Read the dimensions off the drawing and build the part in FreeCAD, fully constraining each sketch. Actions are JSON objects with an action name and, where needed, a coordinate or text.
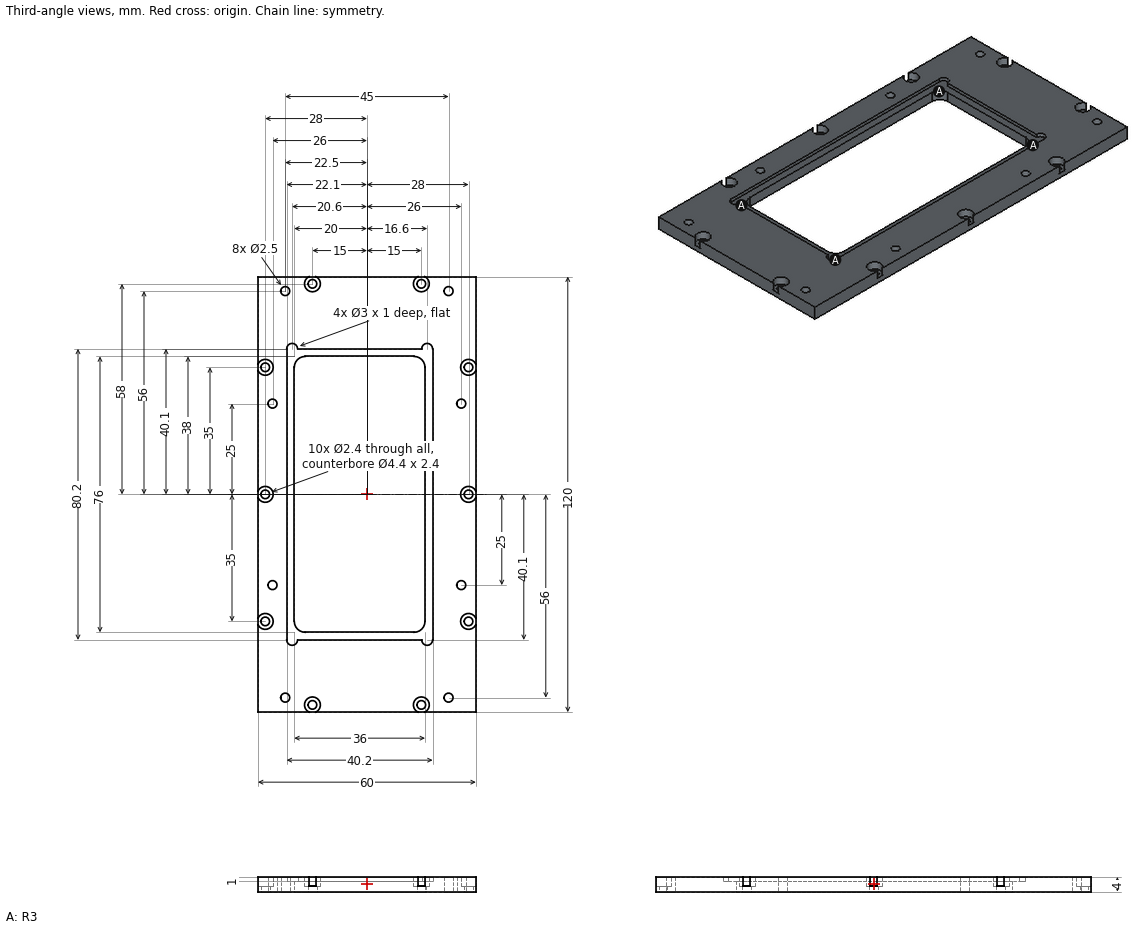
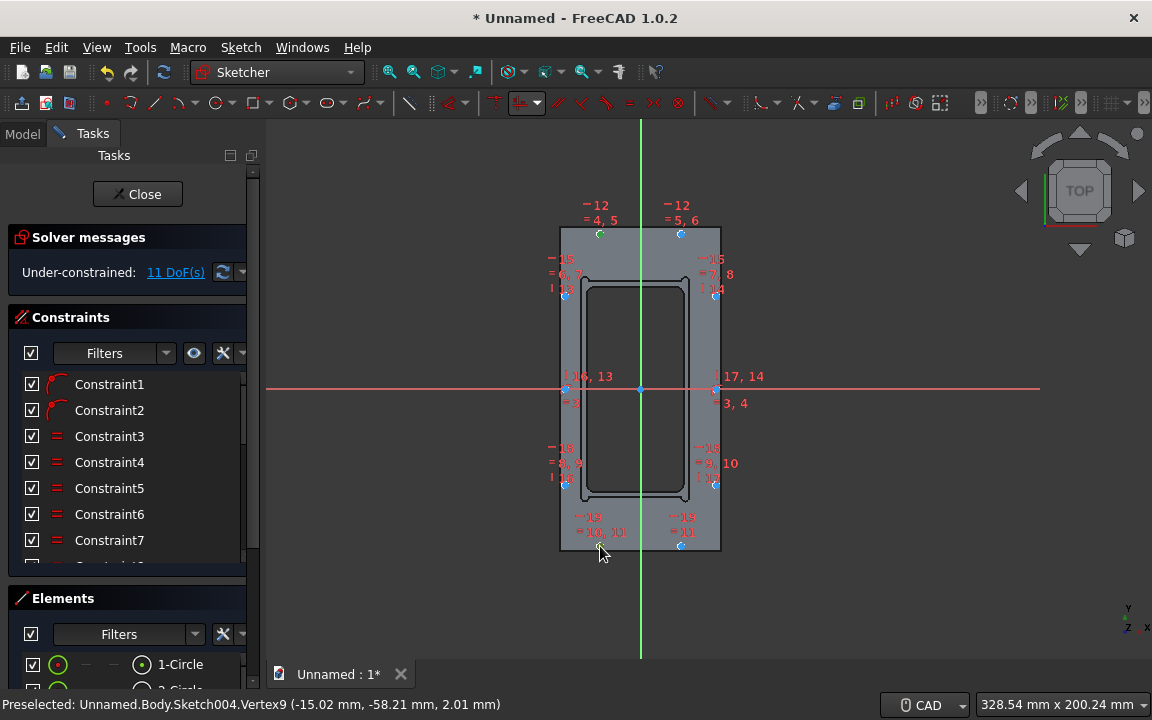
{"action": "left_click", "coordinate": [344, 389]}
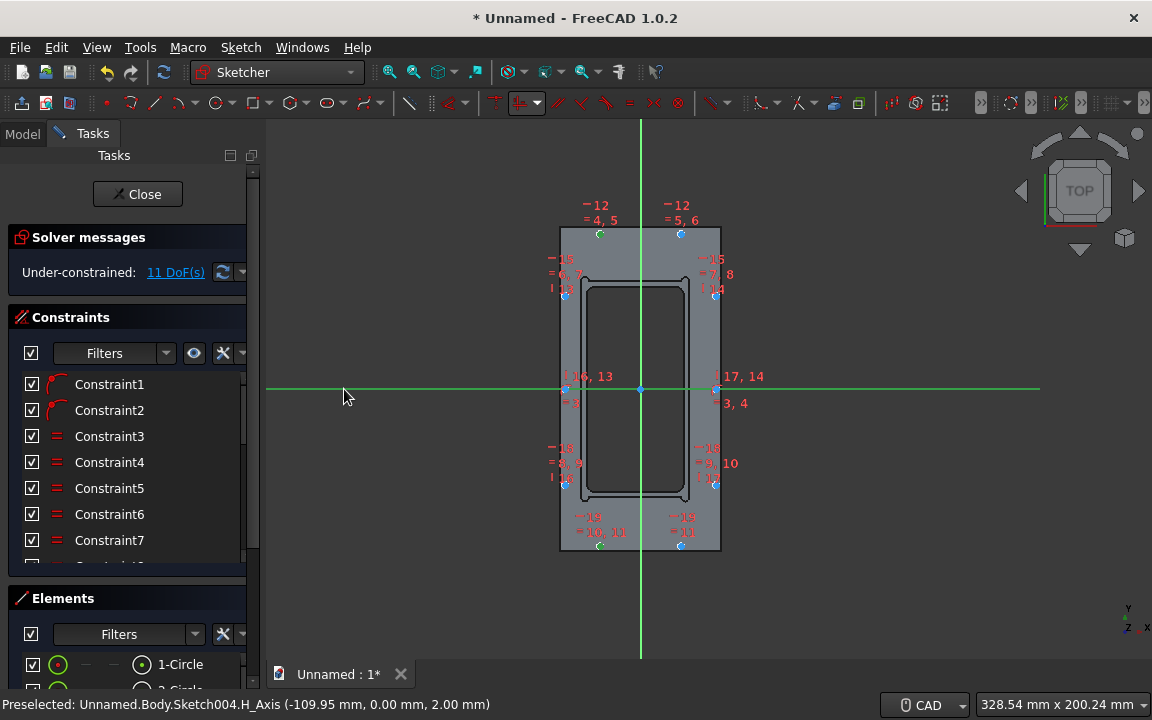
{"action": "key", "text": "s"}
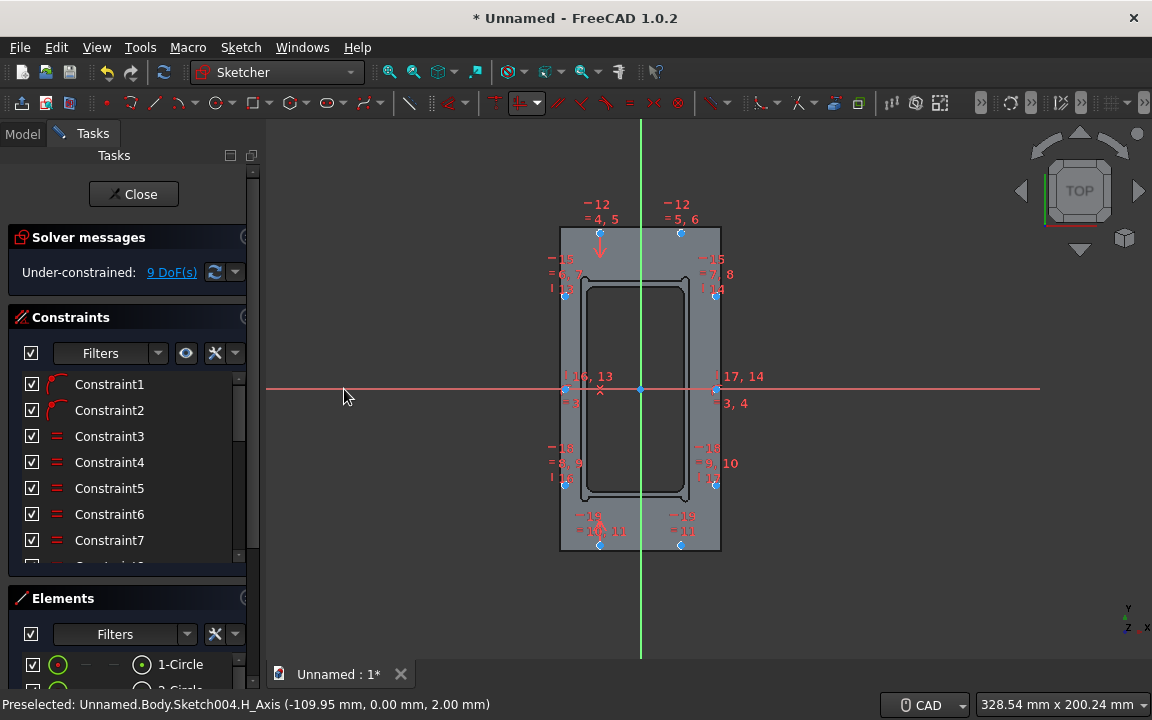
{"action": "key", "text": "d"}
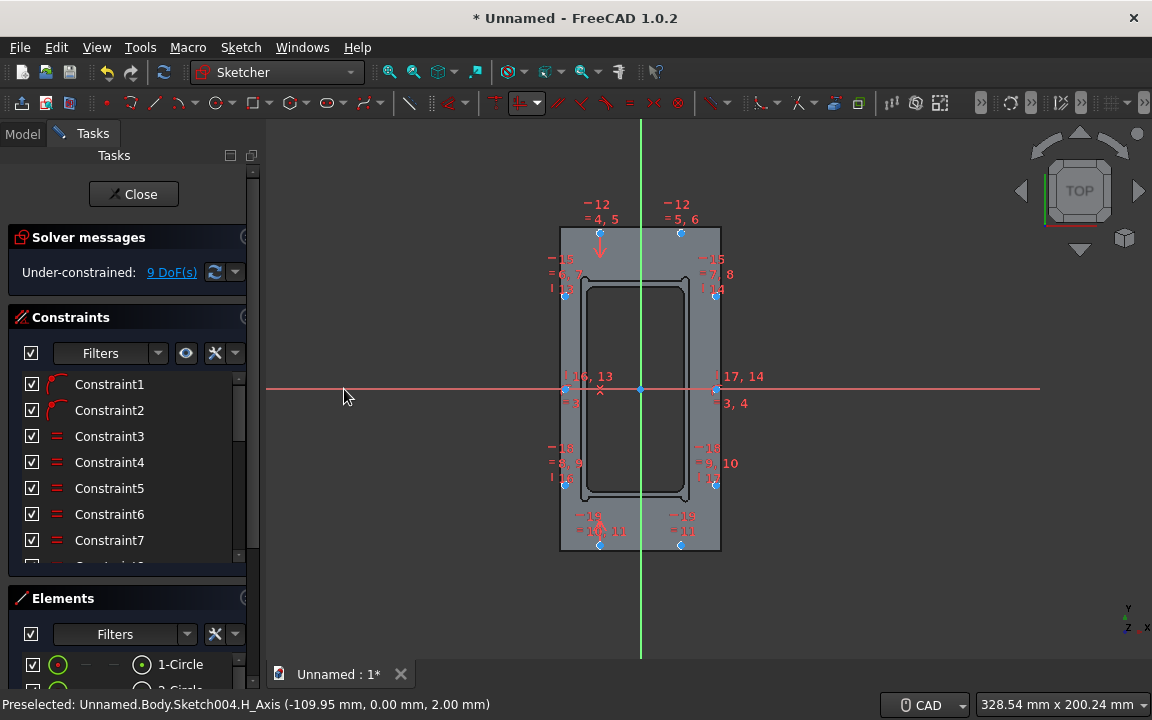
{"action": "scroll", "coordinate": [562, 389], "scroll_direction": "up", "scroll_amount": 10}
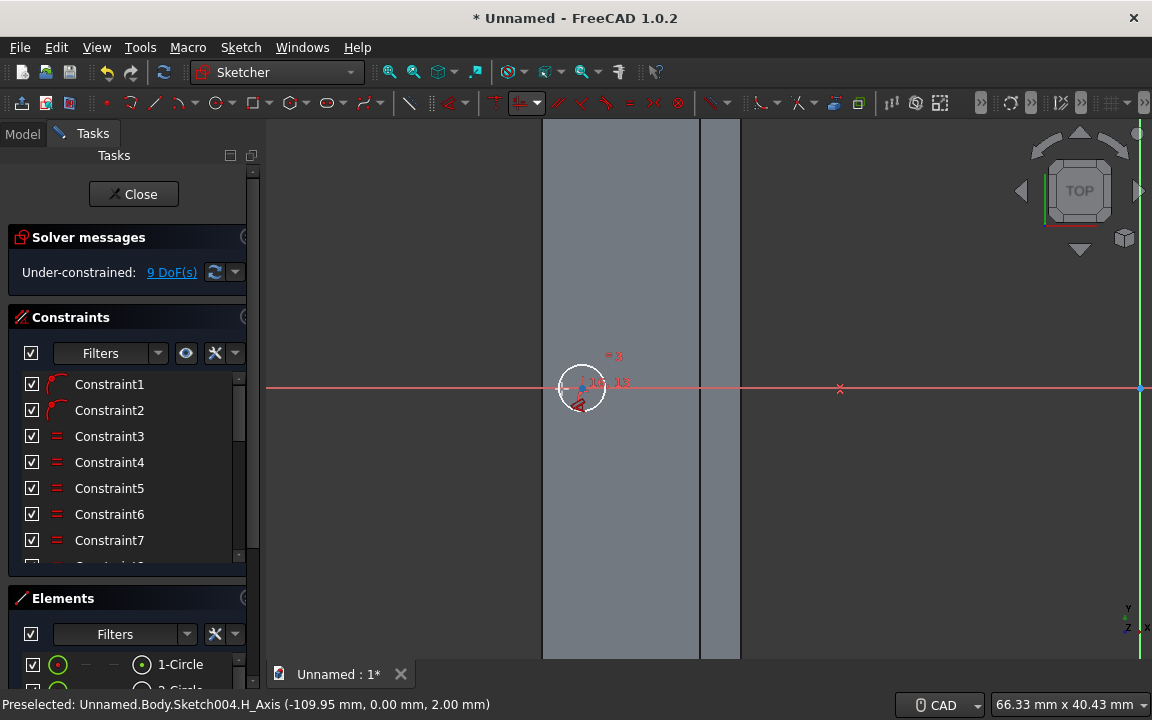
{"action": "left_click", "coordinate": [559, 387]}
{"action": "left_click", "coordinate": [535, 360]}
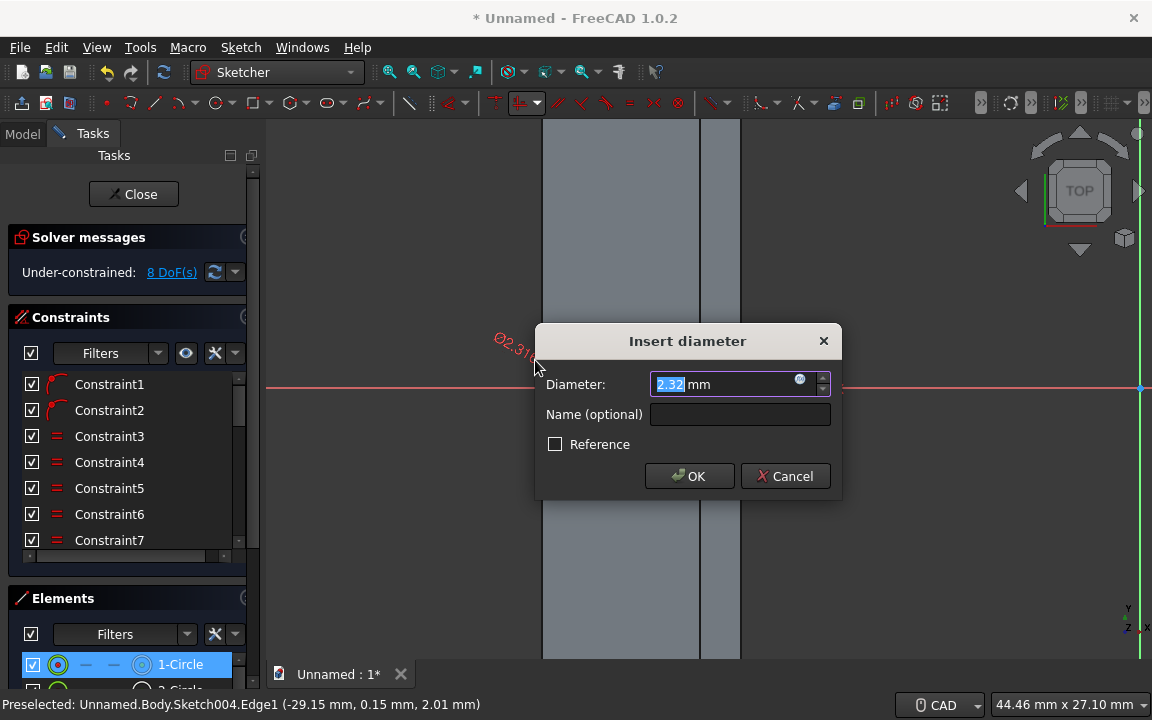
{"action": "type", "text": "2.4"}
{"action": "key", "text": "Return"}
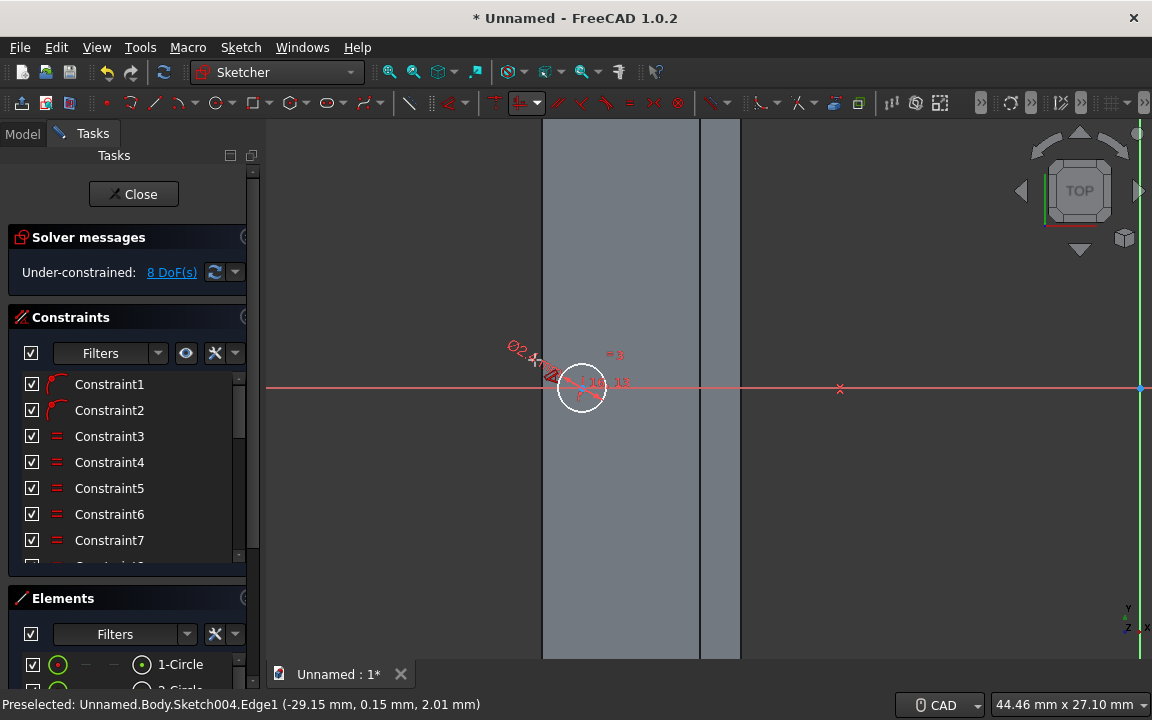
{"action": "scroll", "coordinate": [562, 389], "scroll_direction": "down", "scroll_amount": 10}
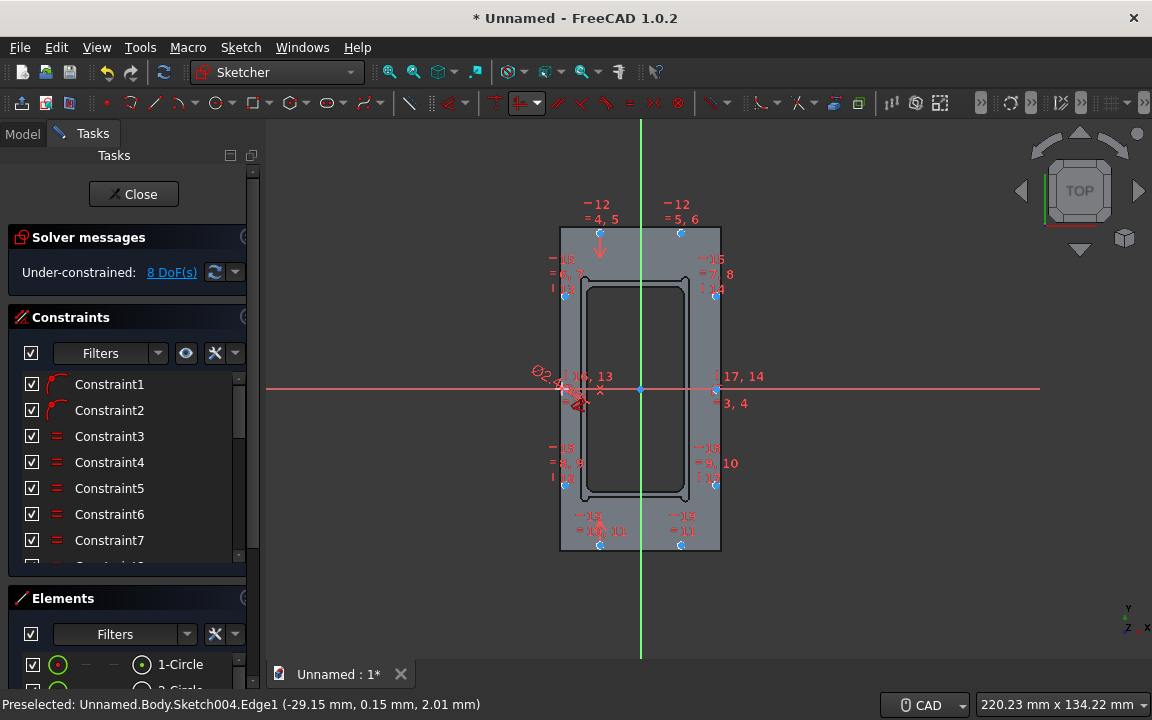
{"action": "left_click", "coordinate": [565, 389]}
{"action": "left_click", "coordinate": [603, 423]}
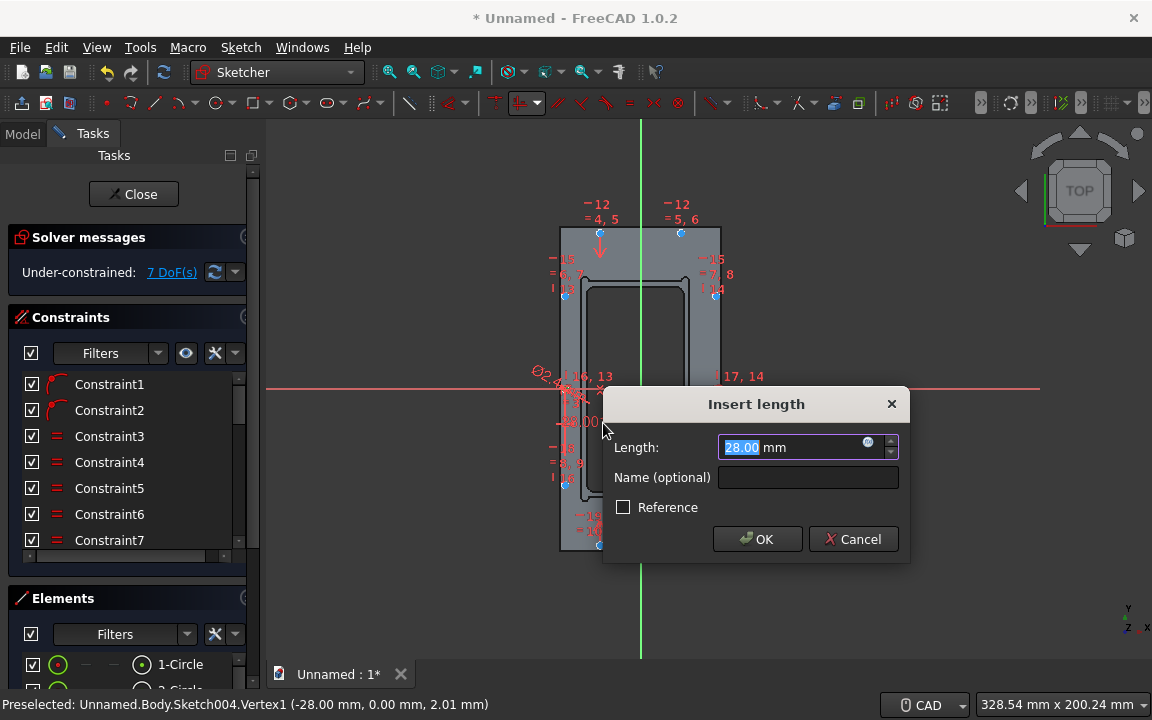
{"action": "type", "text": "28"}
{"action": "key", "text": "Return"}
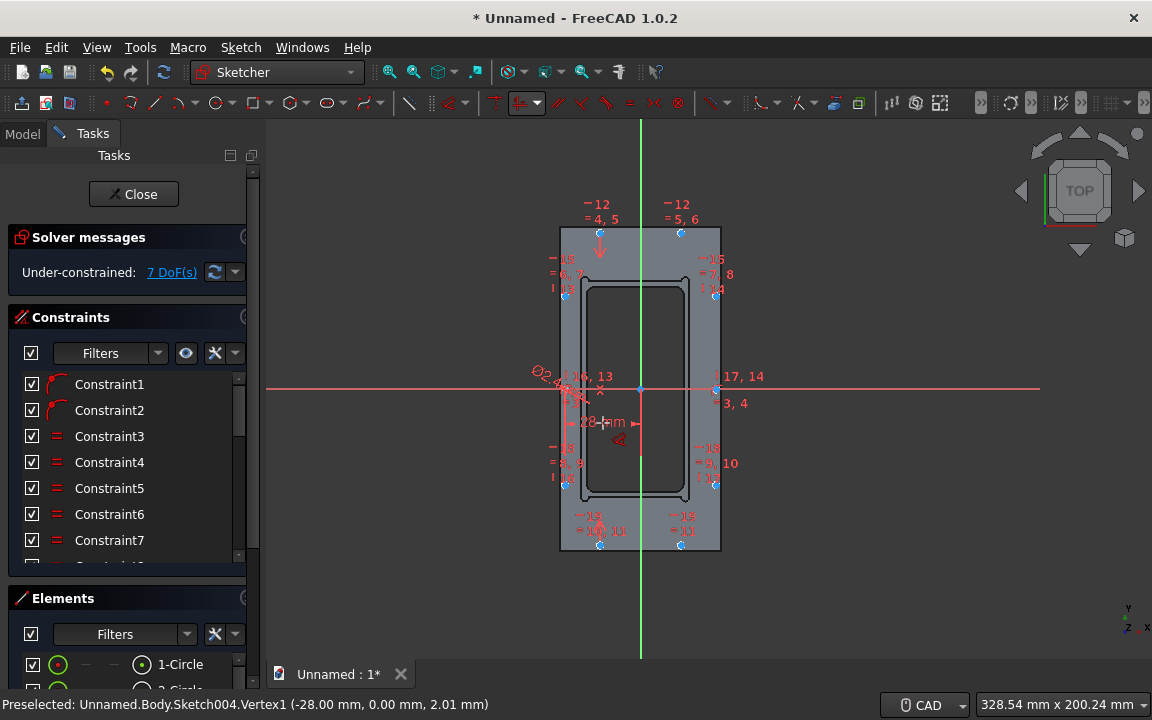
{"action": "left_click", "coordinate": [716, 389]}
{"action": "left_click", "coordinate": [678, 423]}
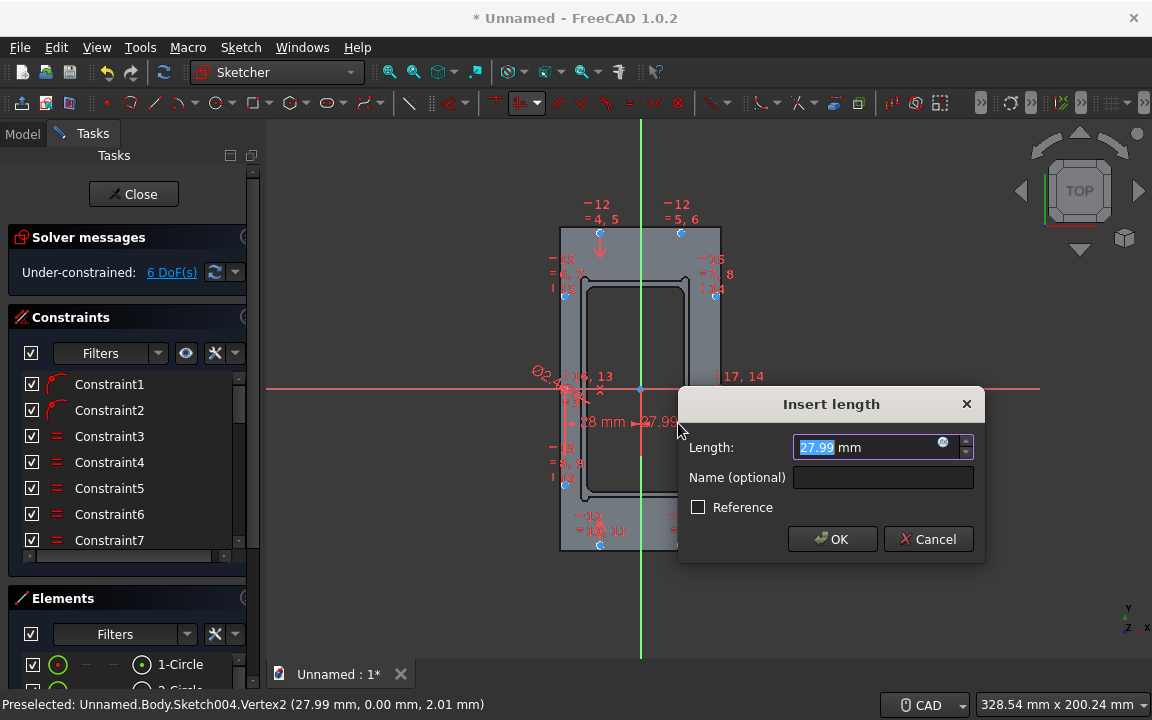
{"action": "type", "text": "28"}
{"action": "key", "text": "Return"}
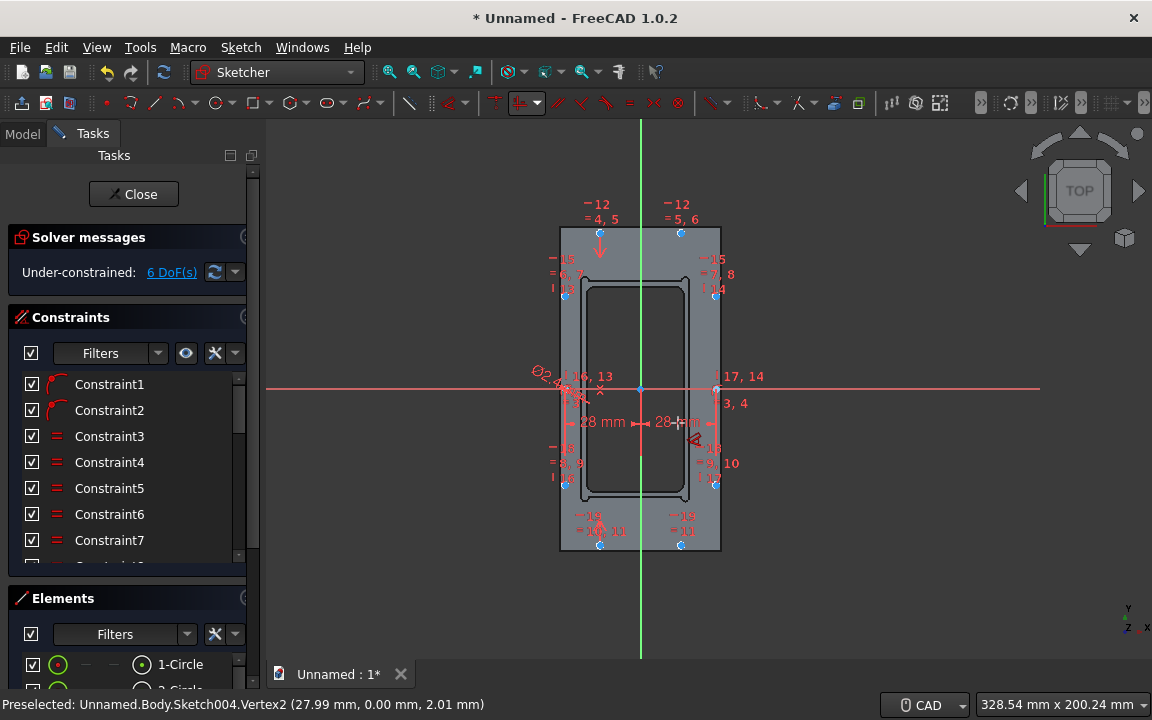
{"action": "left_click", "coordinate": [600, 233]}
{"action": "left_click", "coordinate": [620, 199]}